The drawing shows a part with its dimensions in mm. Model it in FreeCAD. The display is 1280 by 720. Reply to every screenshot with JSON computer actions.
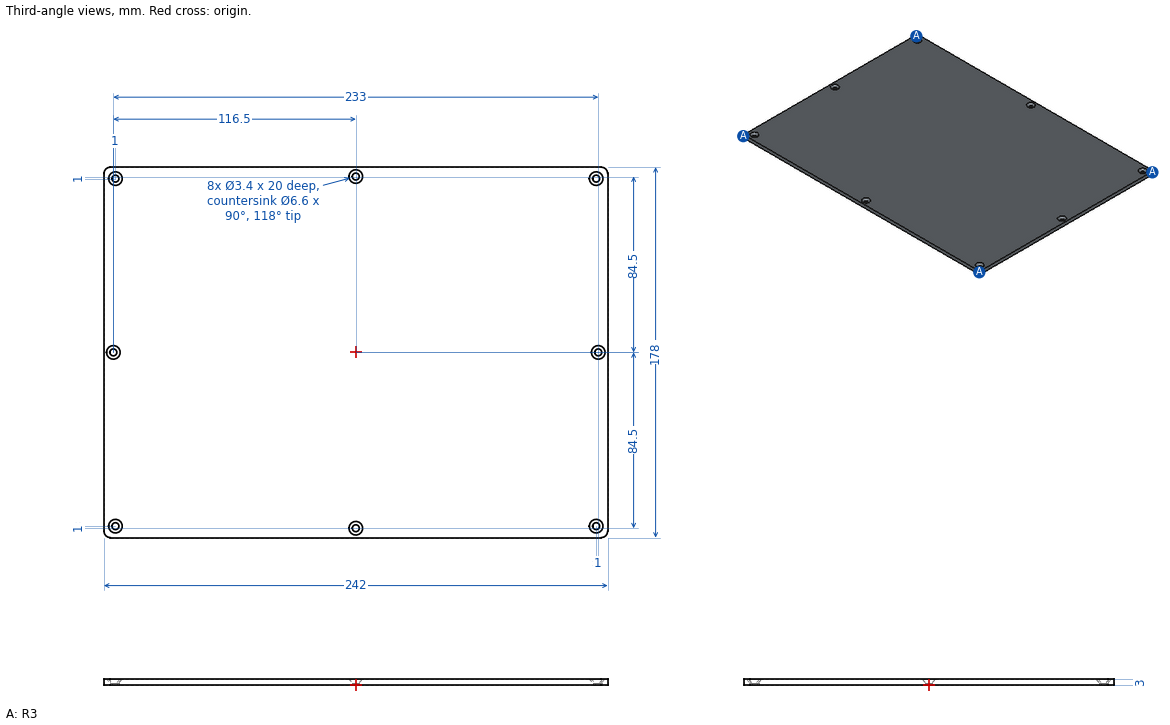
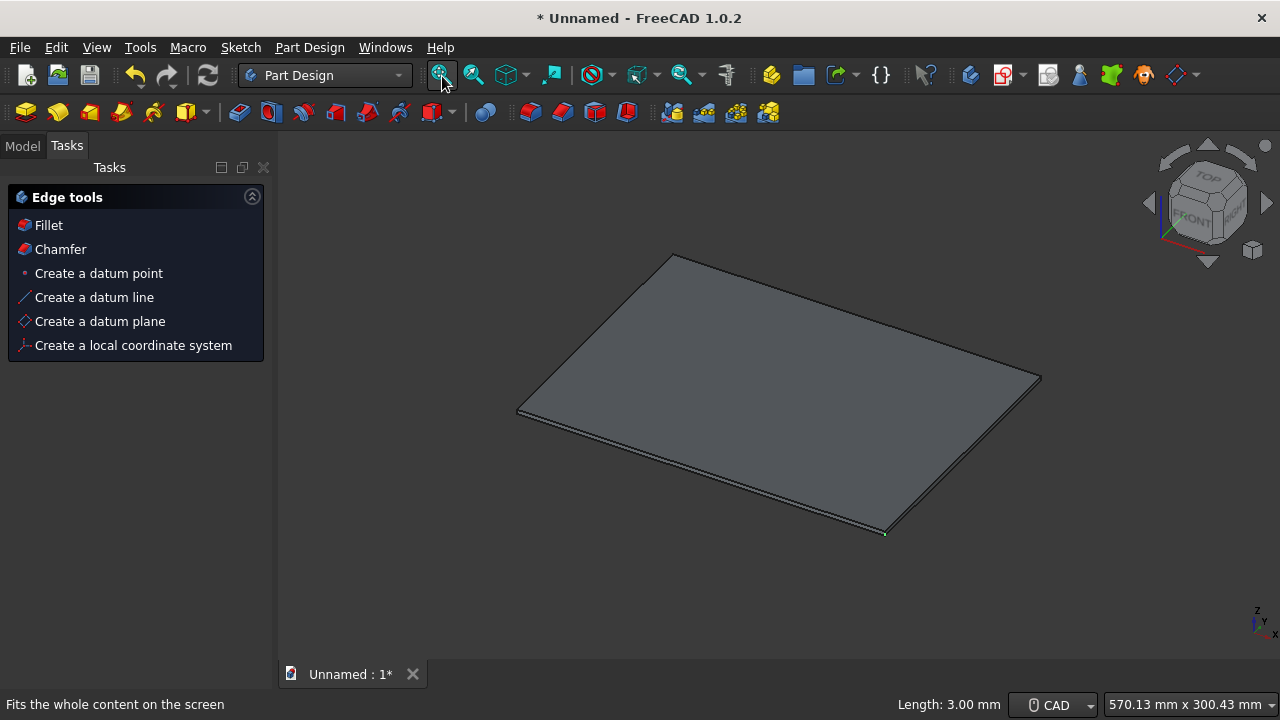
{"action": "key", "text": "0"}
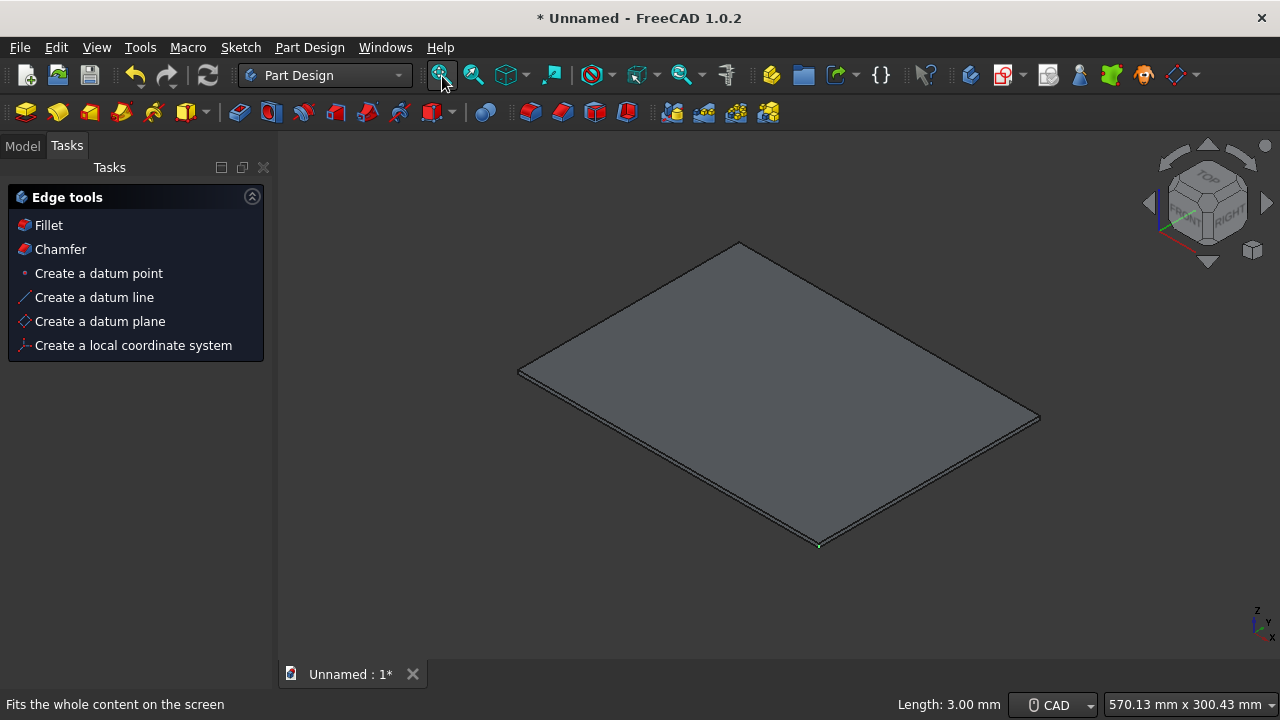
{"action": "scroll", "coordinate": [518, 371], "scroll_direction": "up", "scroll_amount": 11}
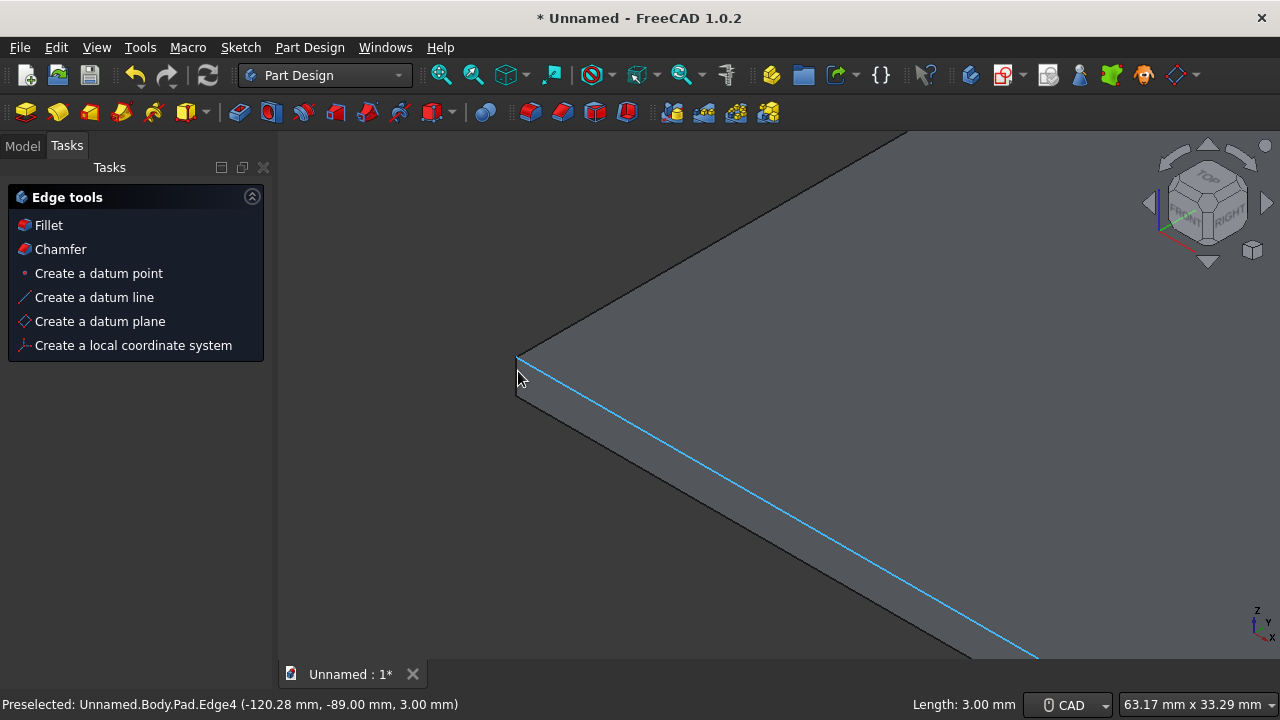
{"action": "left_click", "coordinate": [442, 76]}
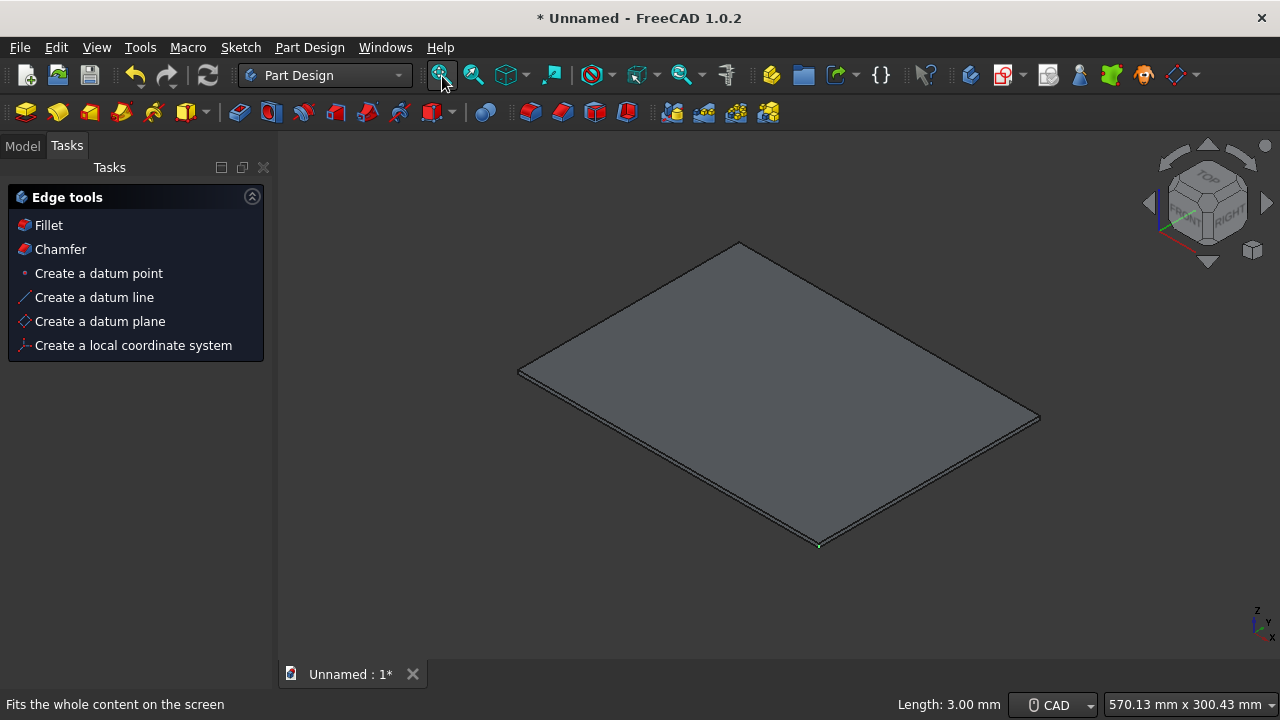
{"action": "key", "text": "2"}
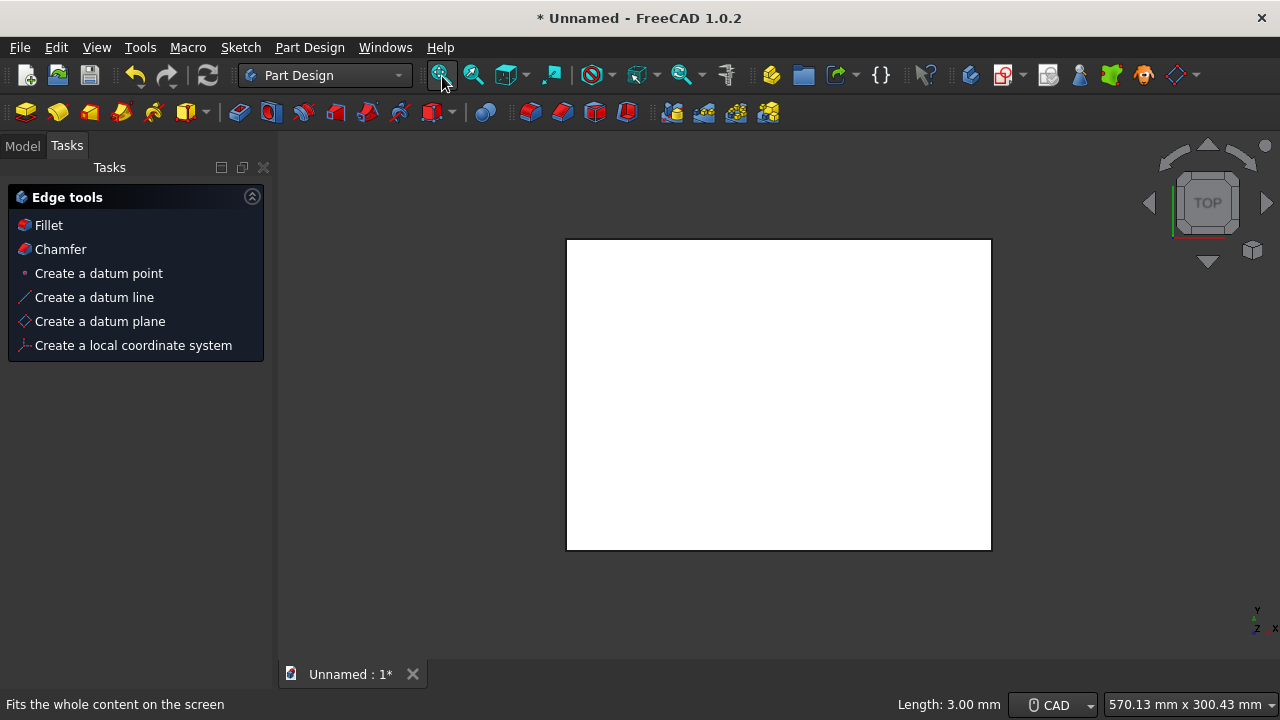
{"action": "scroll", "coordinate": [566, 550], "scroll_direction": "up", "scroll_amount": 11}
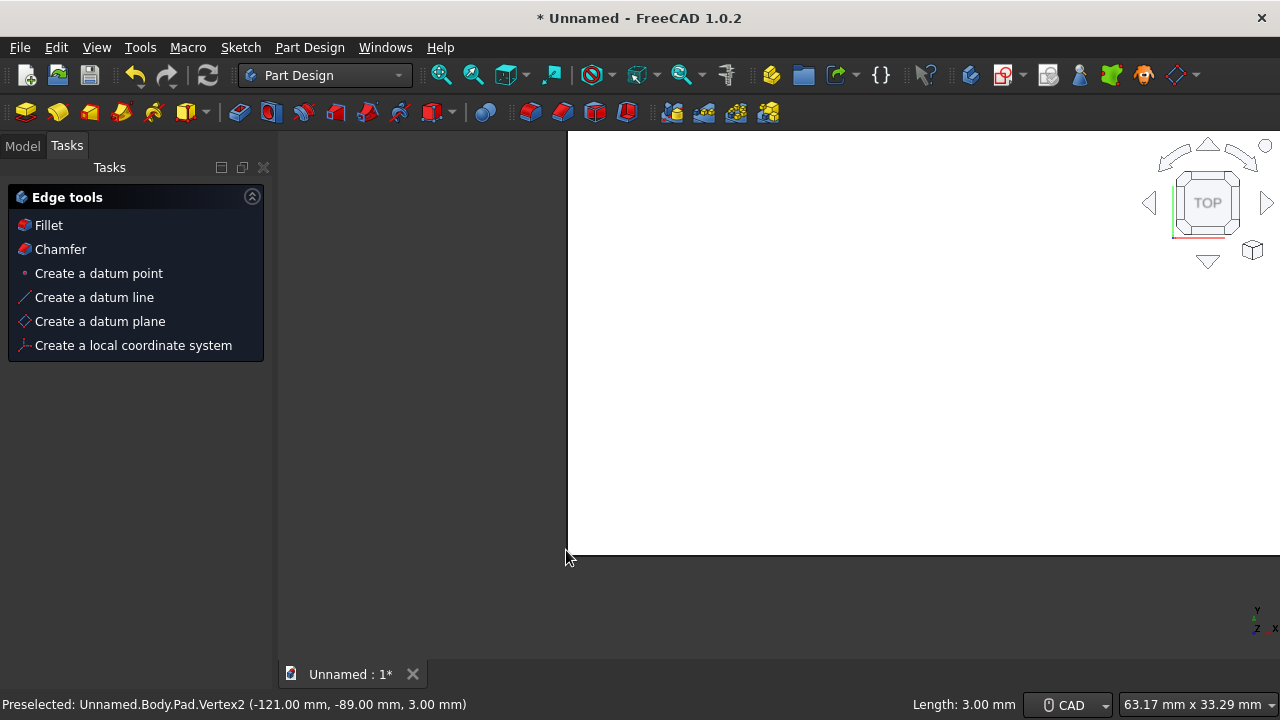
{"action": "left_click", "coordinate": [442, 76]}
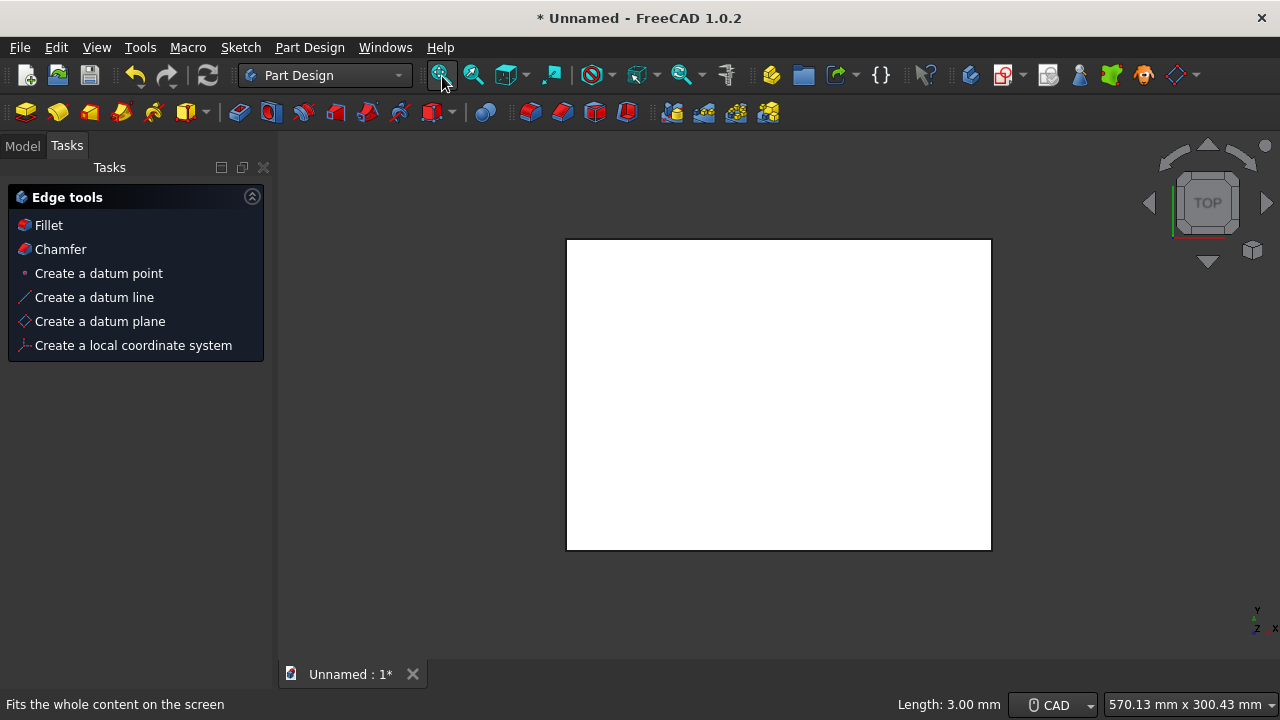
{"action": "key", "text": "1"}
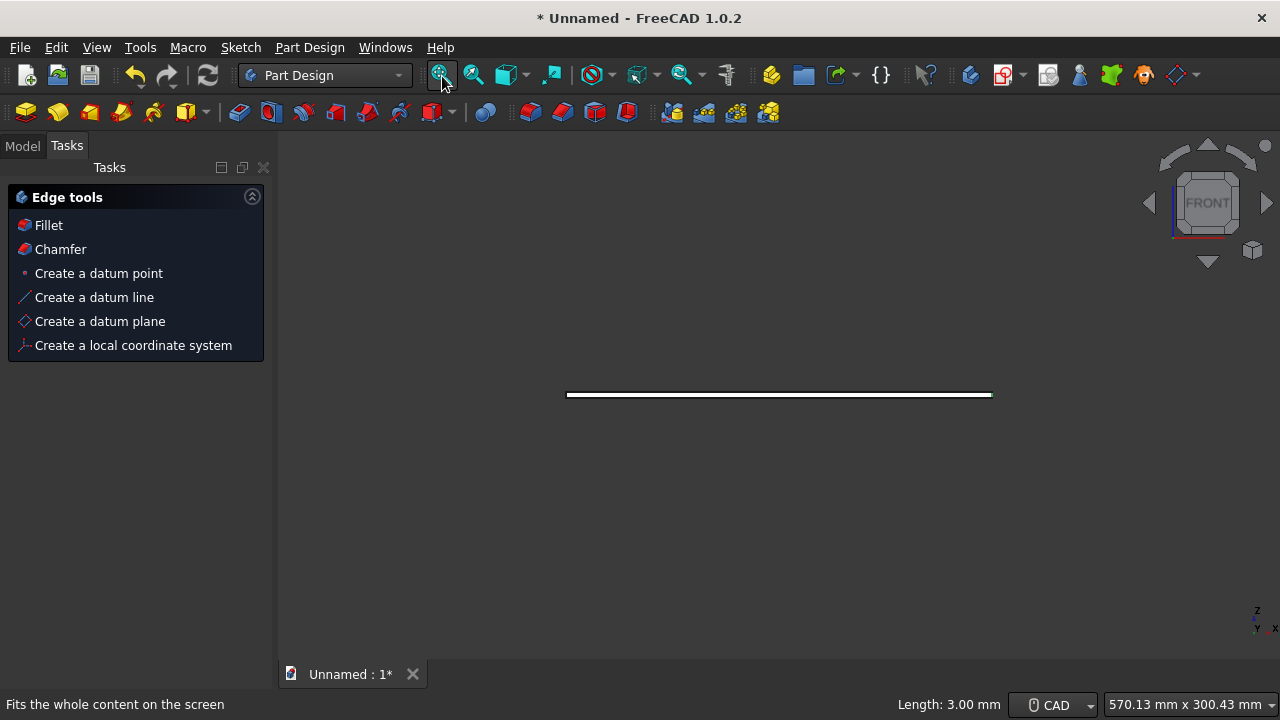
{"action": "left_click", "coordinate": [442, 76]}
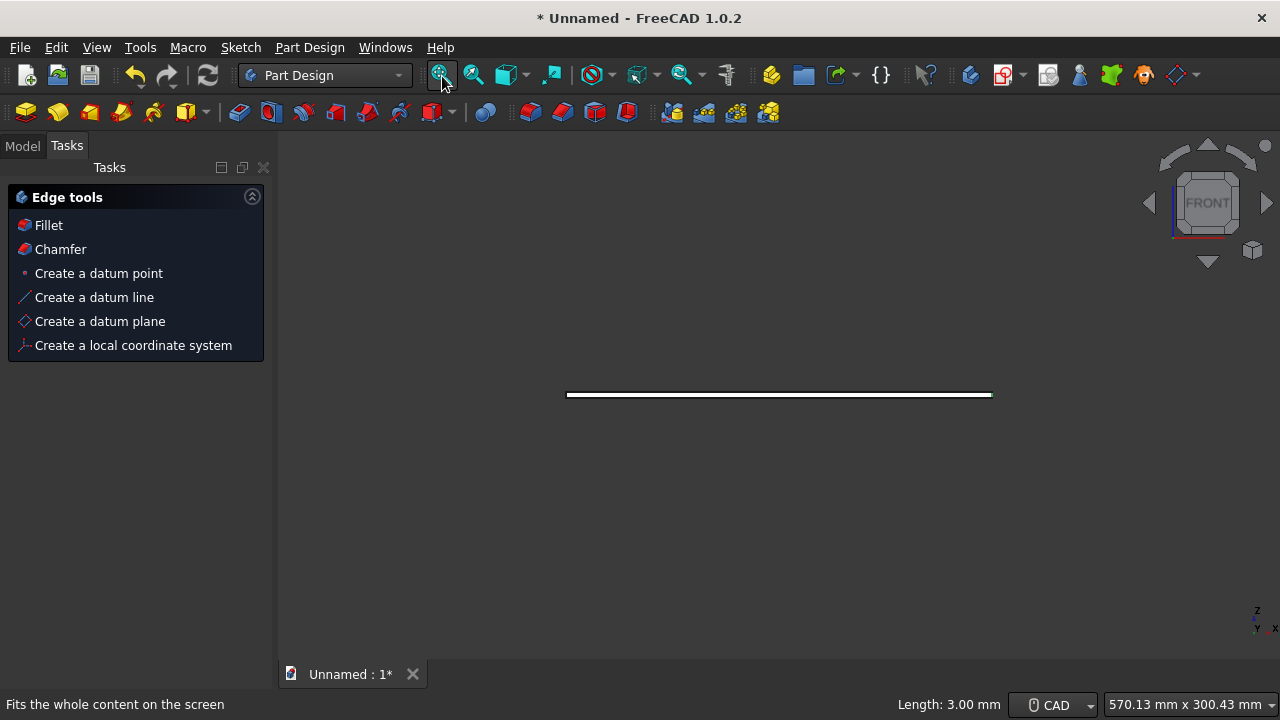
{"action": "scroll", "coordinate": [566, 394], "scroll_direction": "up", "scroll_amount": 11}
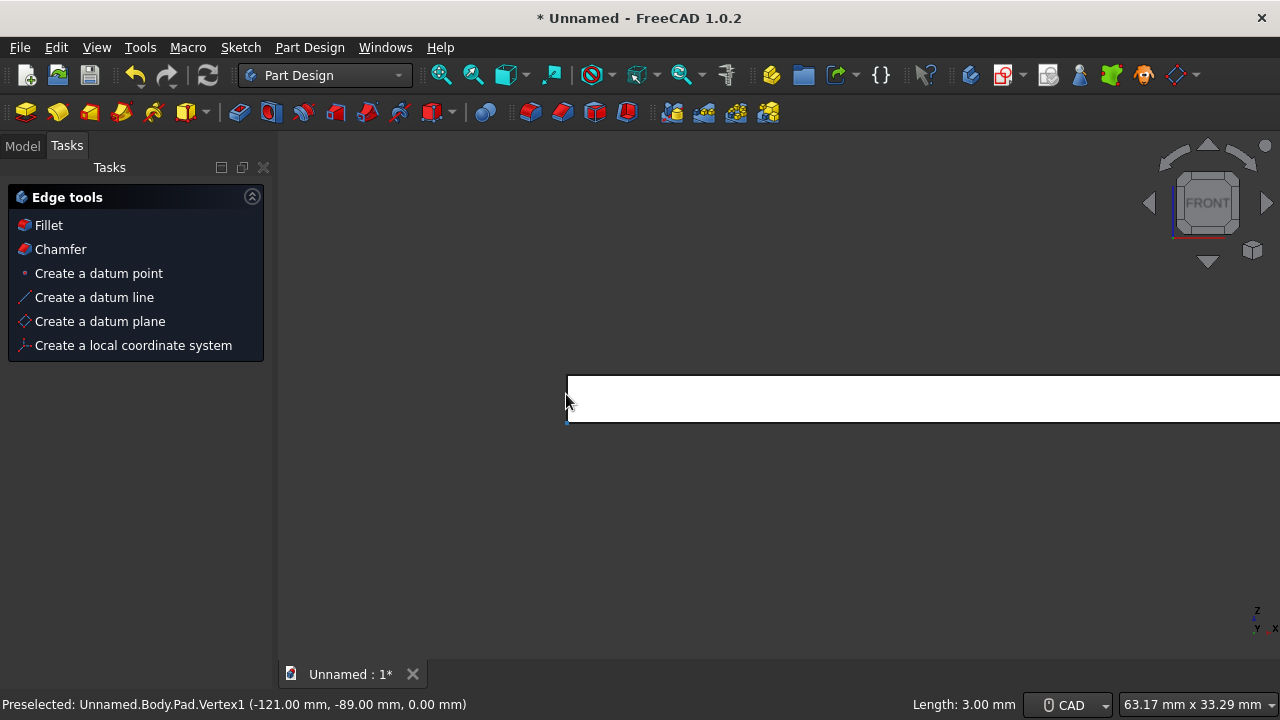
{"action": "left_click", "coordinate": [567, 398], "text": "ctrl"}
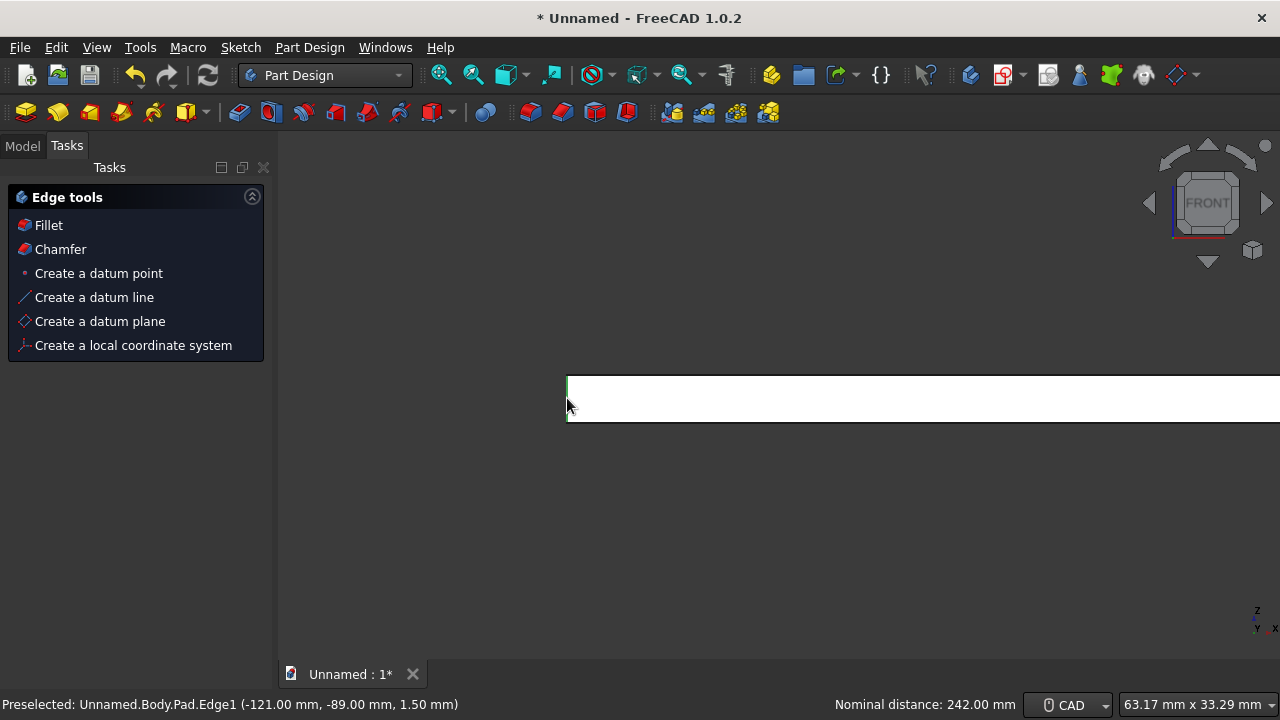
{"action": "left_click", "coordinate": [442, 76]}